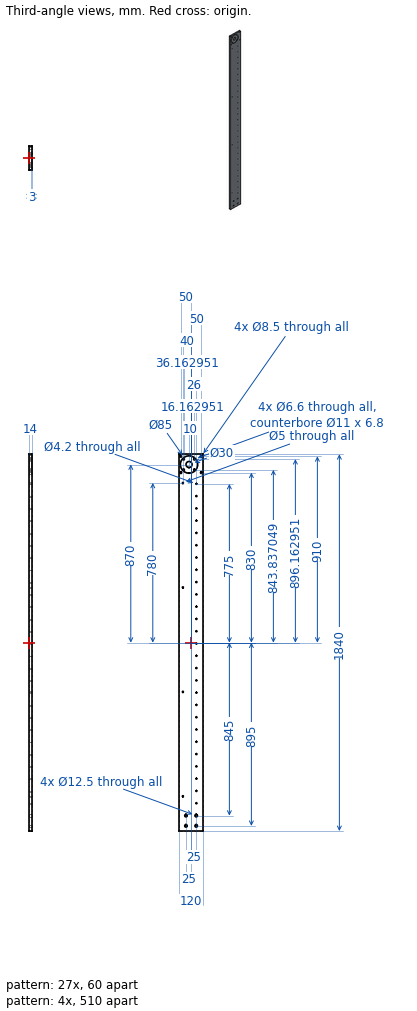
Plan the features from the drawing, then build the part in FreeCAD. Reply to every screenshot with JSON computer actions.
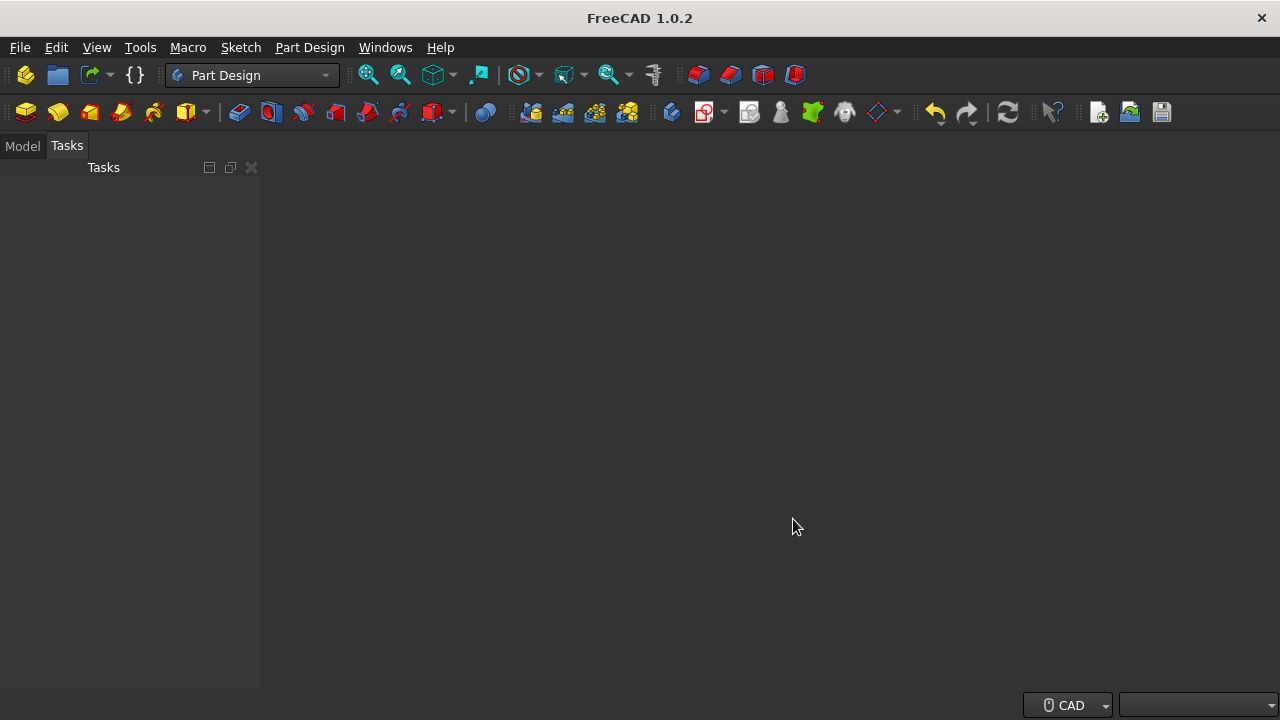
{"action": "left_click", "coordinate": [1098, 112]}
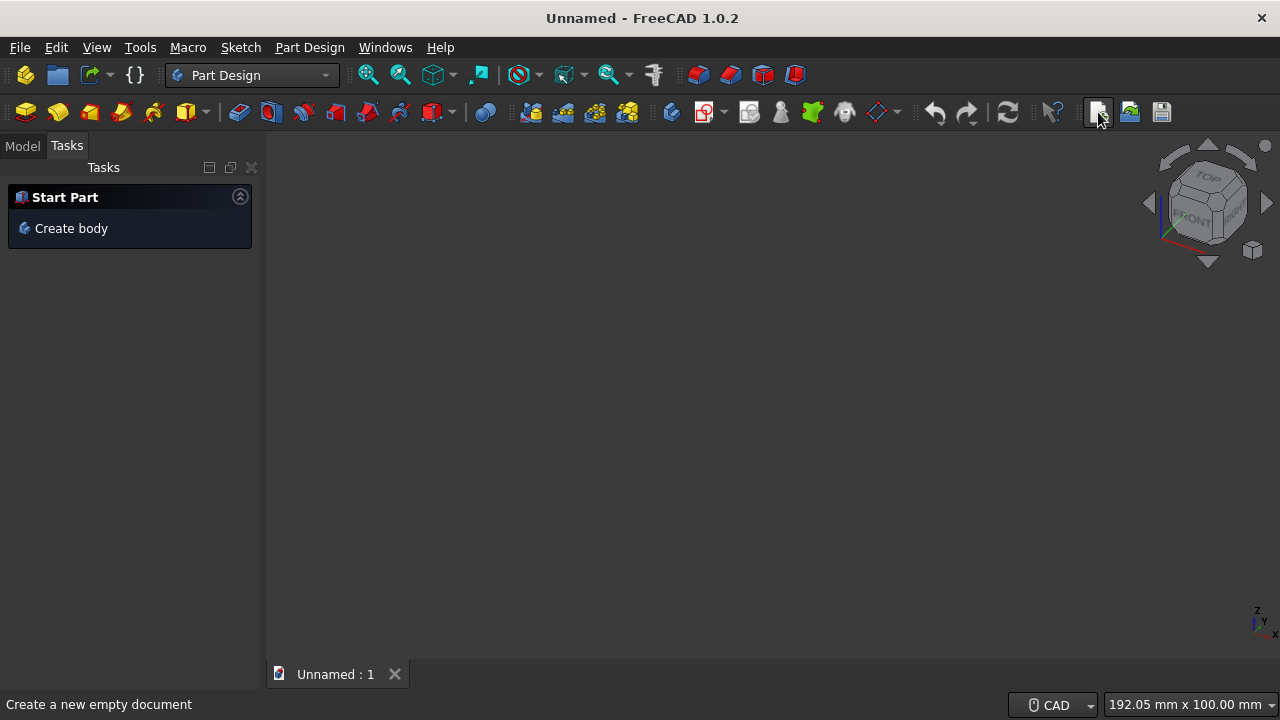
{"action": "left_click", "coordinate": [704, 112]}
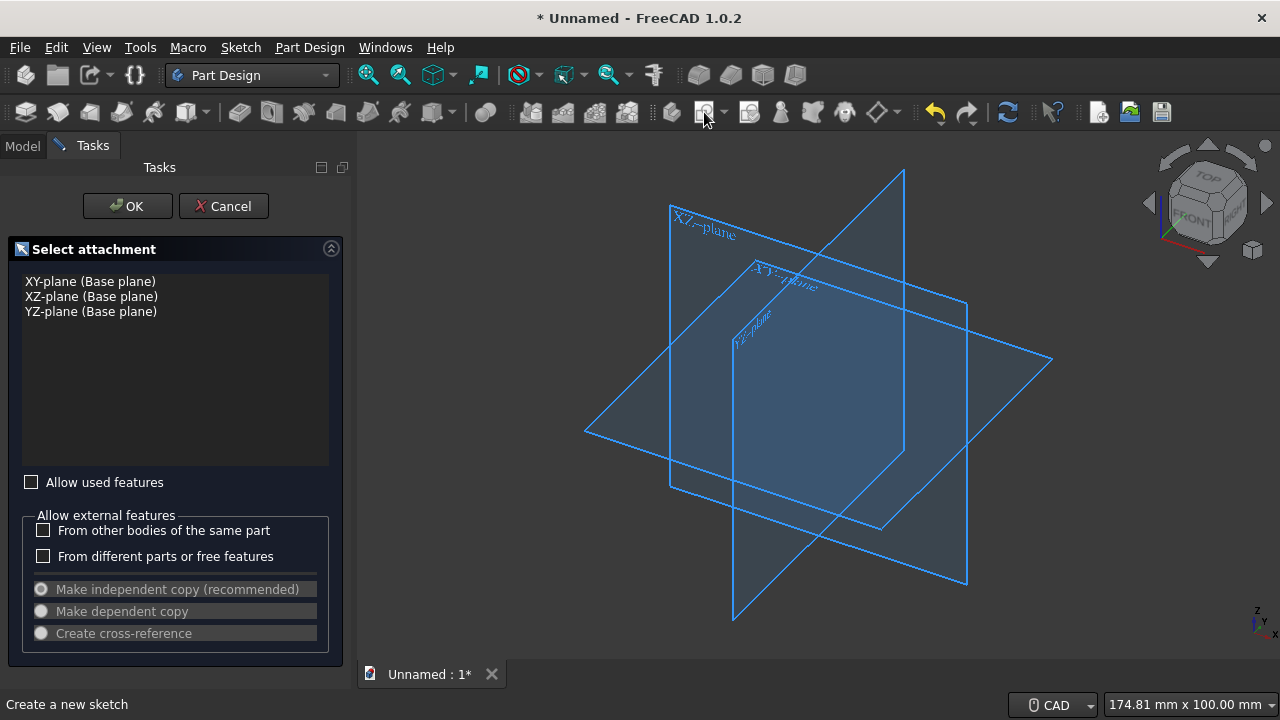
{"action": "left_click", "coordinate": [82, 312]}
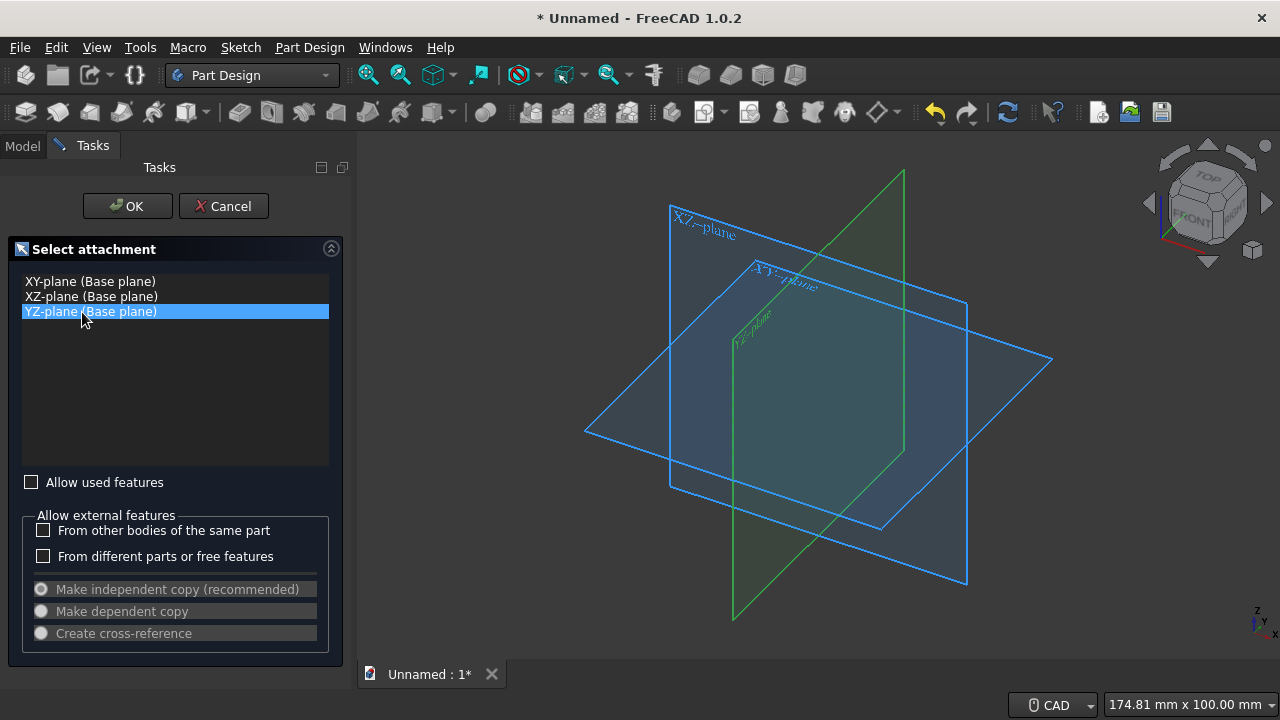
{"action": "left_click", "coordinate": [128, 206]}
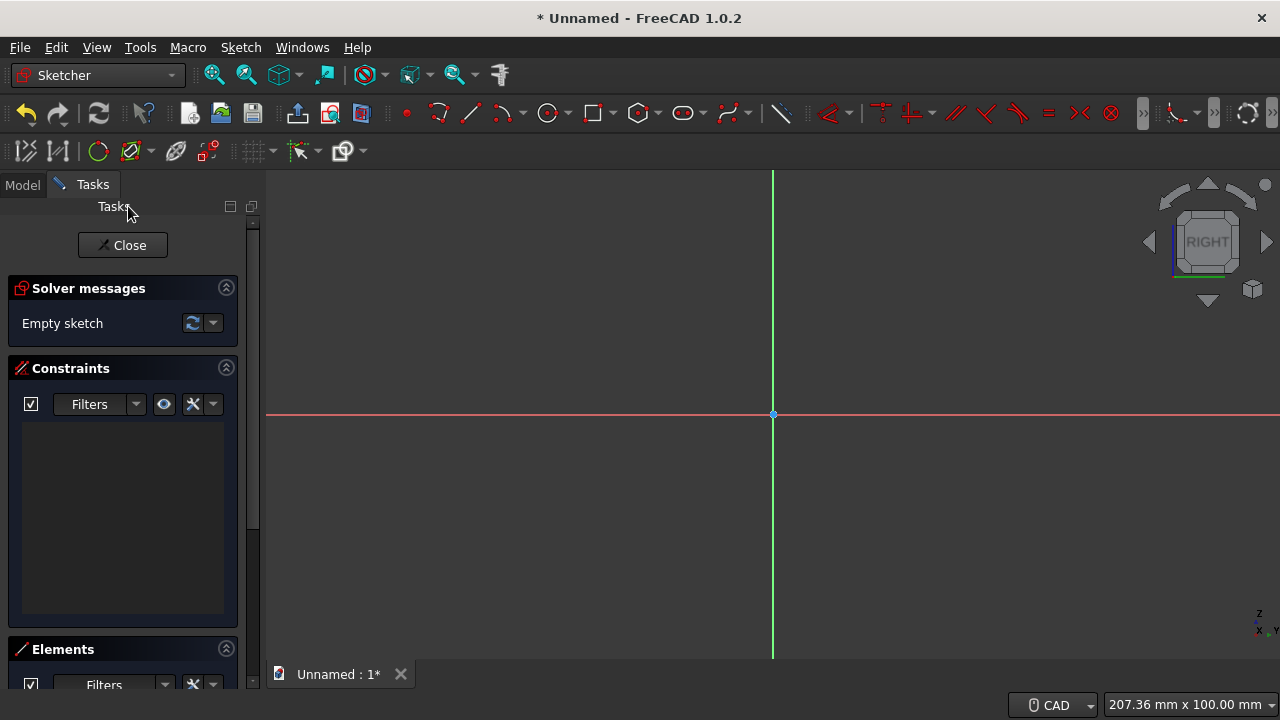
{"action": "scroll", "coordinate": [702, 414], "scroll_direction": "down", "scroll_amount": 16}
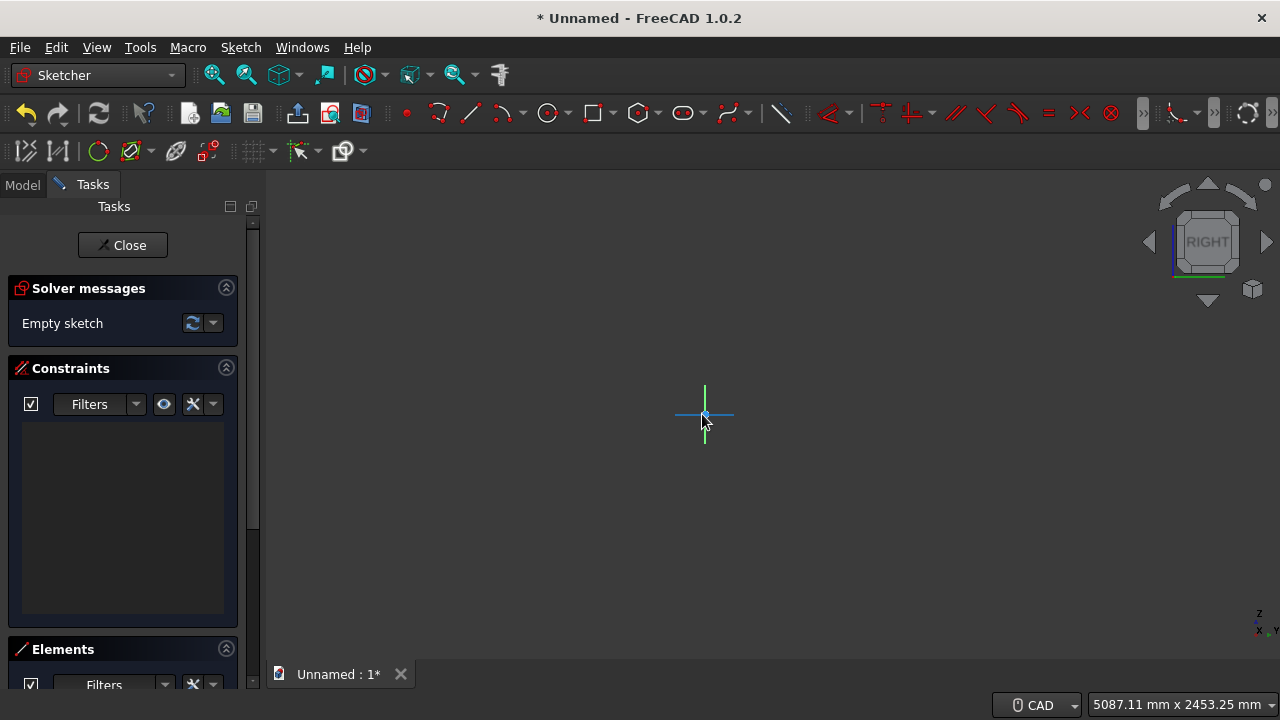
{"action": "left_click", "coordinate": [616, 114]}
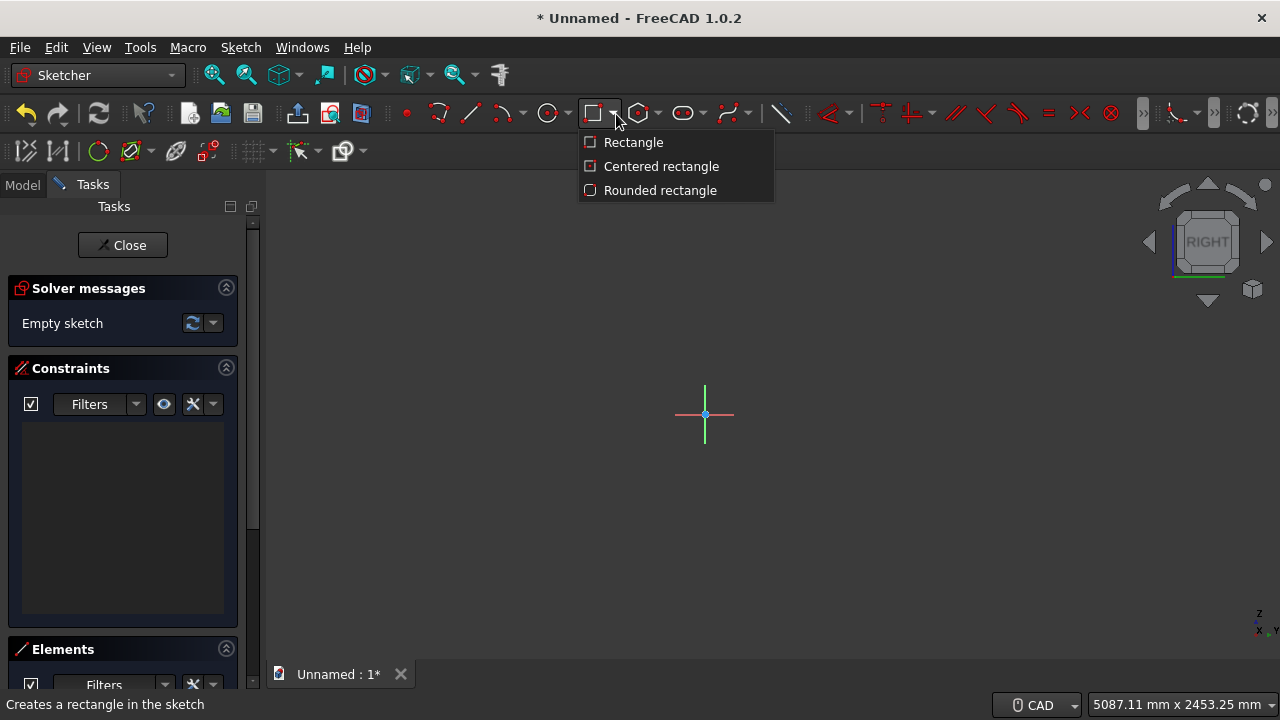
{"action": "left_click", "coordinate": [676, 166]}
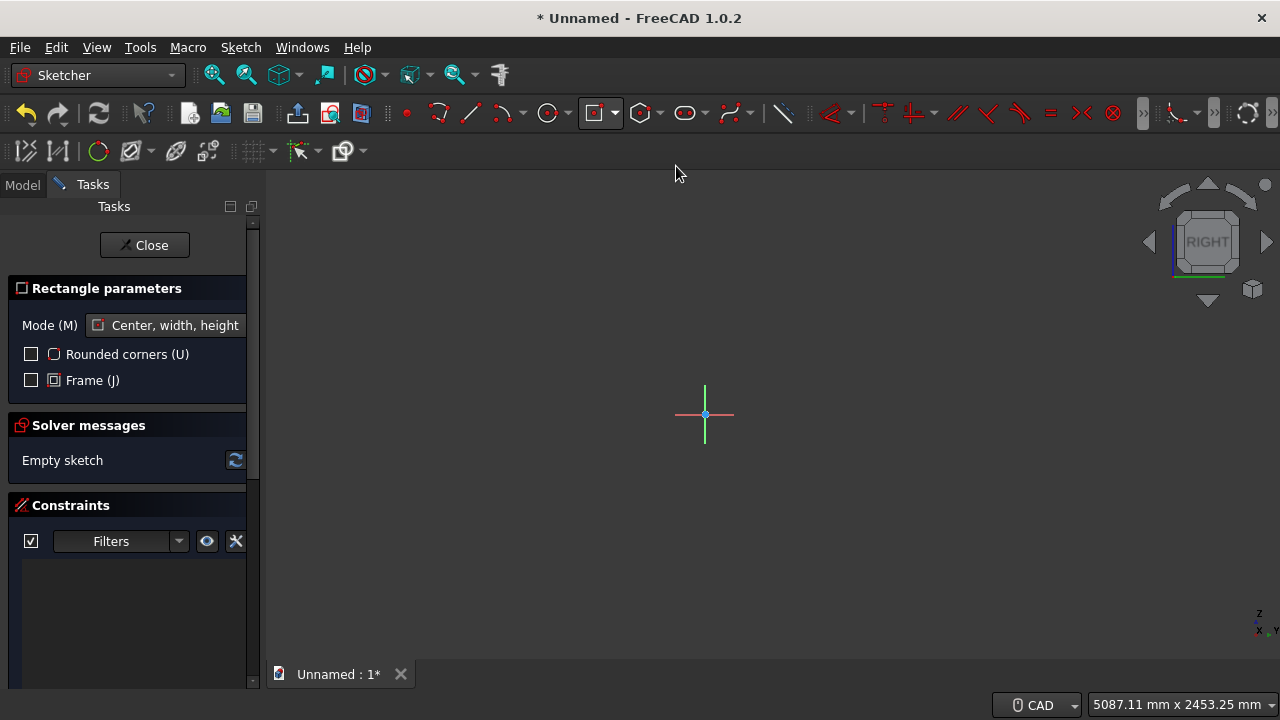
{"action": "scroll", "coordinate": [705, 414], "scroll_direction": "up", "scroll_amount": 2}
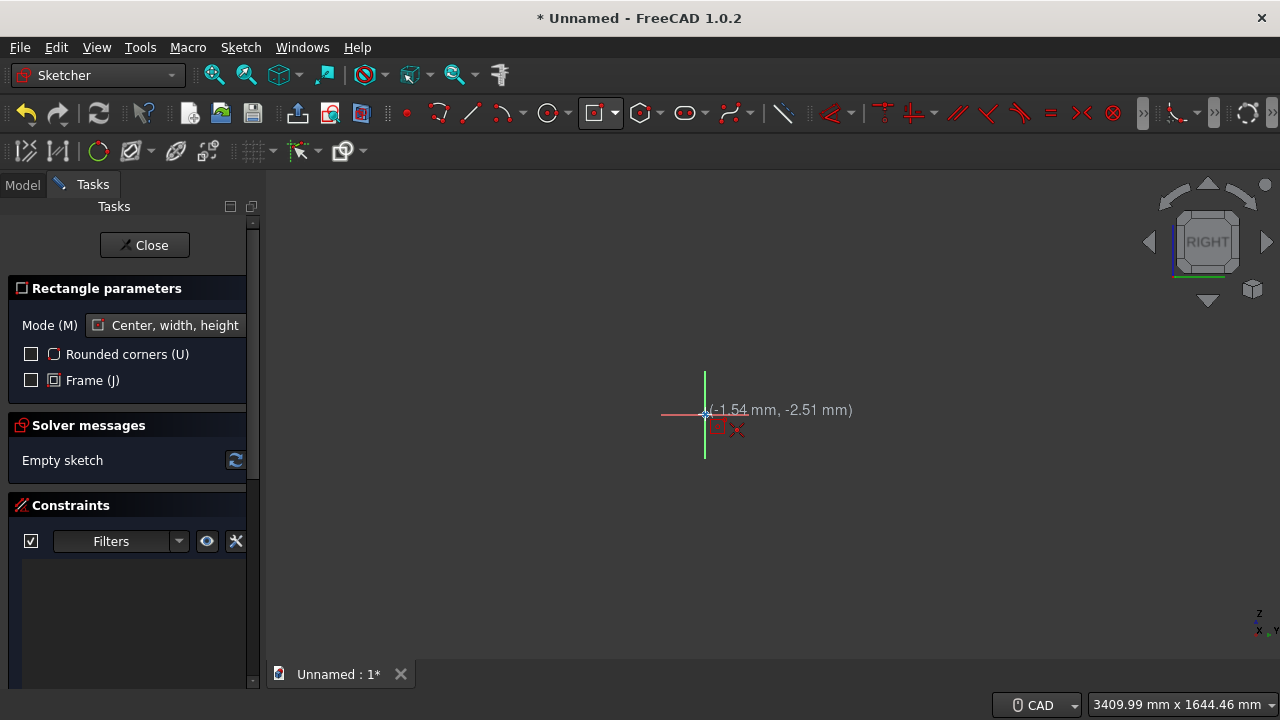
{"action": "left_click", "coordinate": [705, 414]}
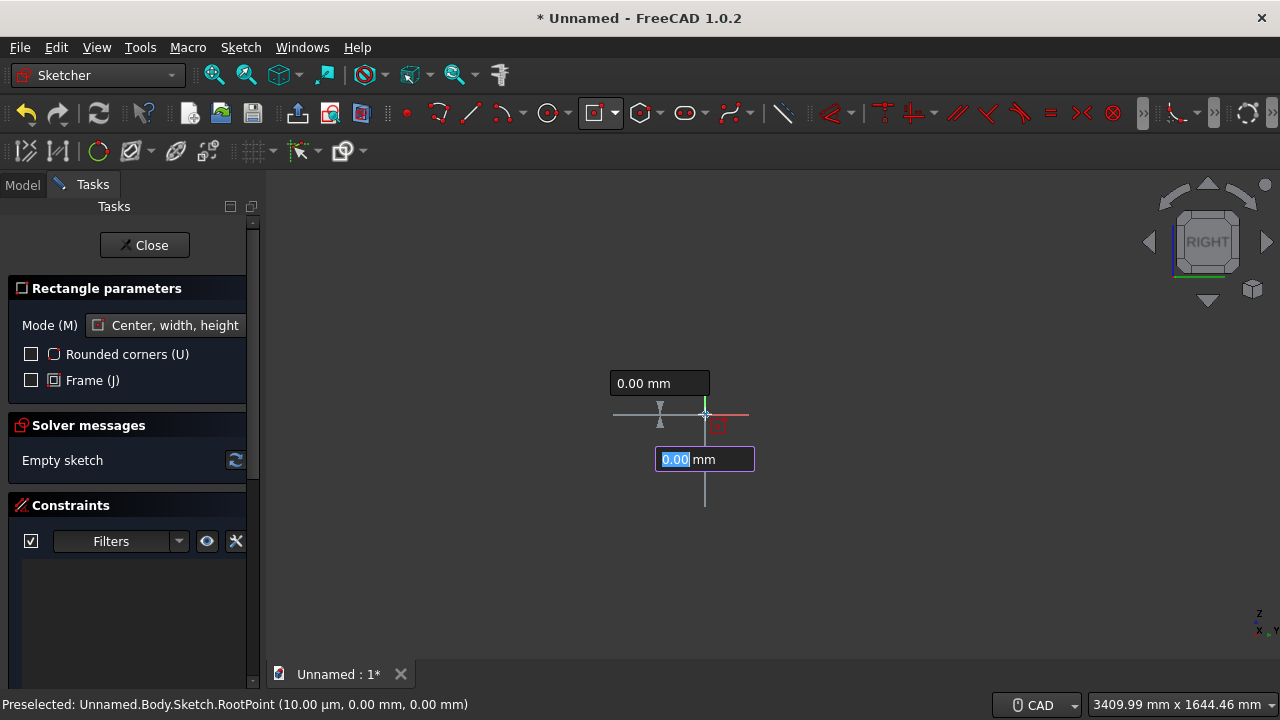
{"action": "scroll", "coordinate": [704, 414], "scroll_direction": "down", "scroll_amount": 3}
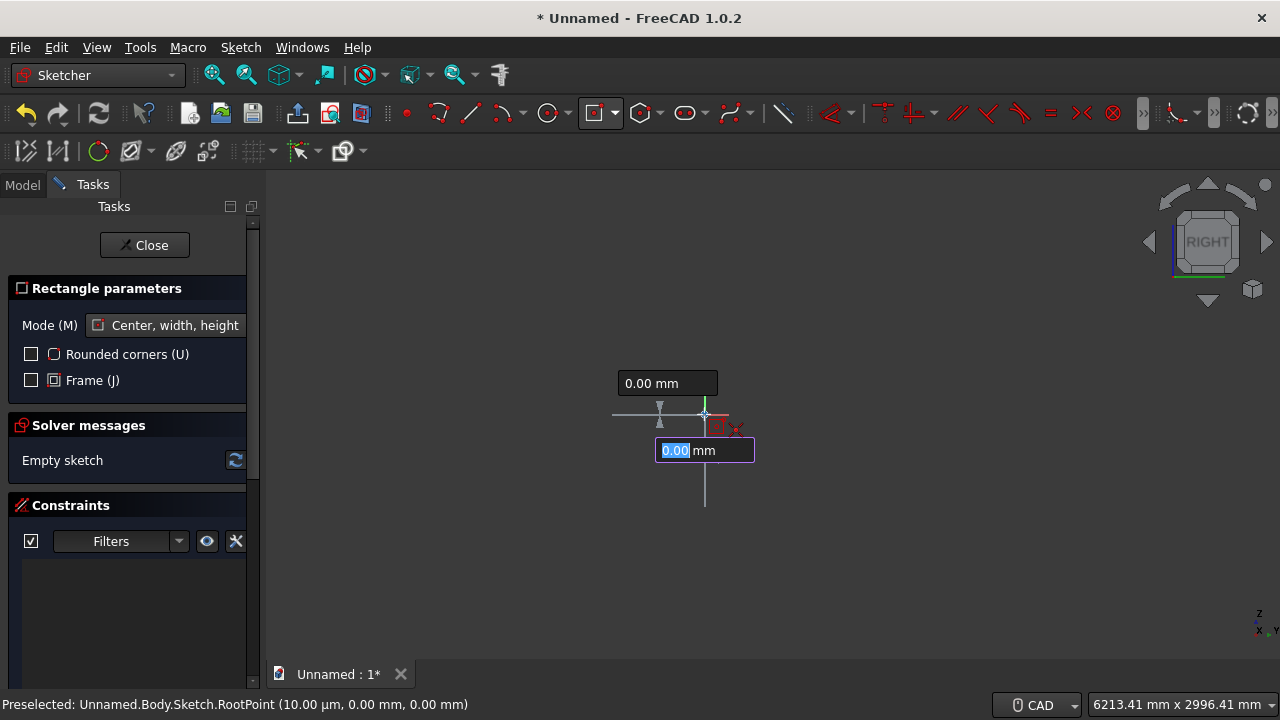
{"action": "scroll", "coordinate": [715, 264], "scroll_direction": "up", "scroll_amount": 3}